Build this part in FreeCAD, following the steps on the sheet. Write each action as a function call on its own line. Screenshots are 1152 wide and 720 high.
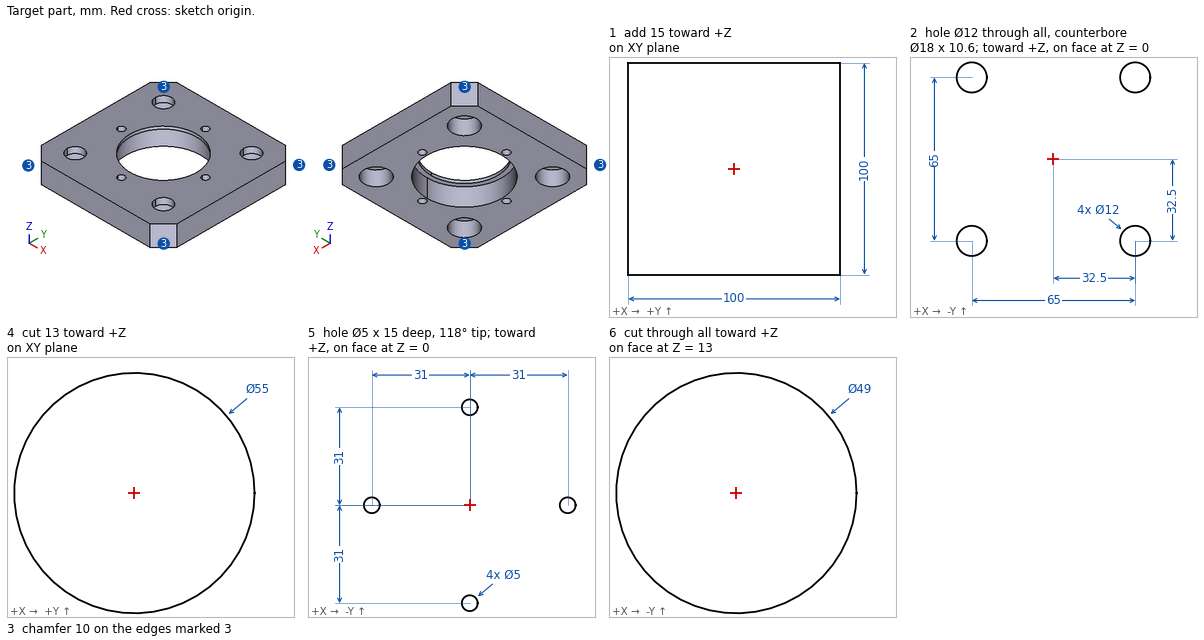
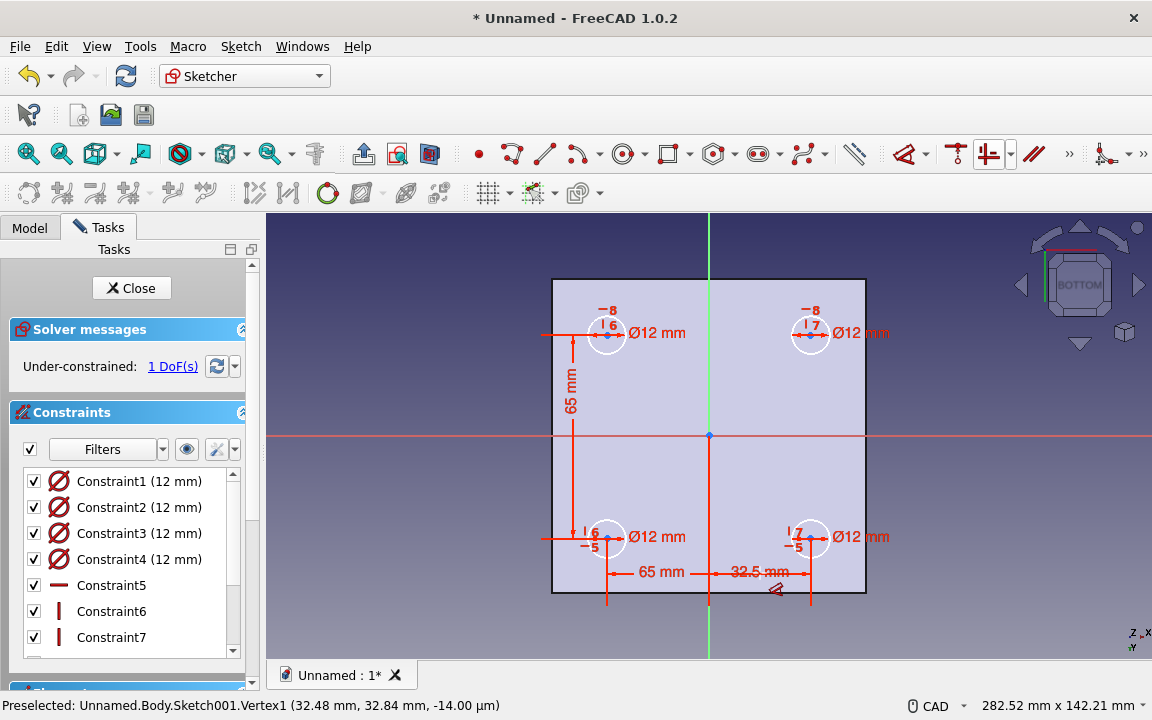
click(811, 539)
click(845, 487)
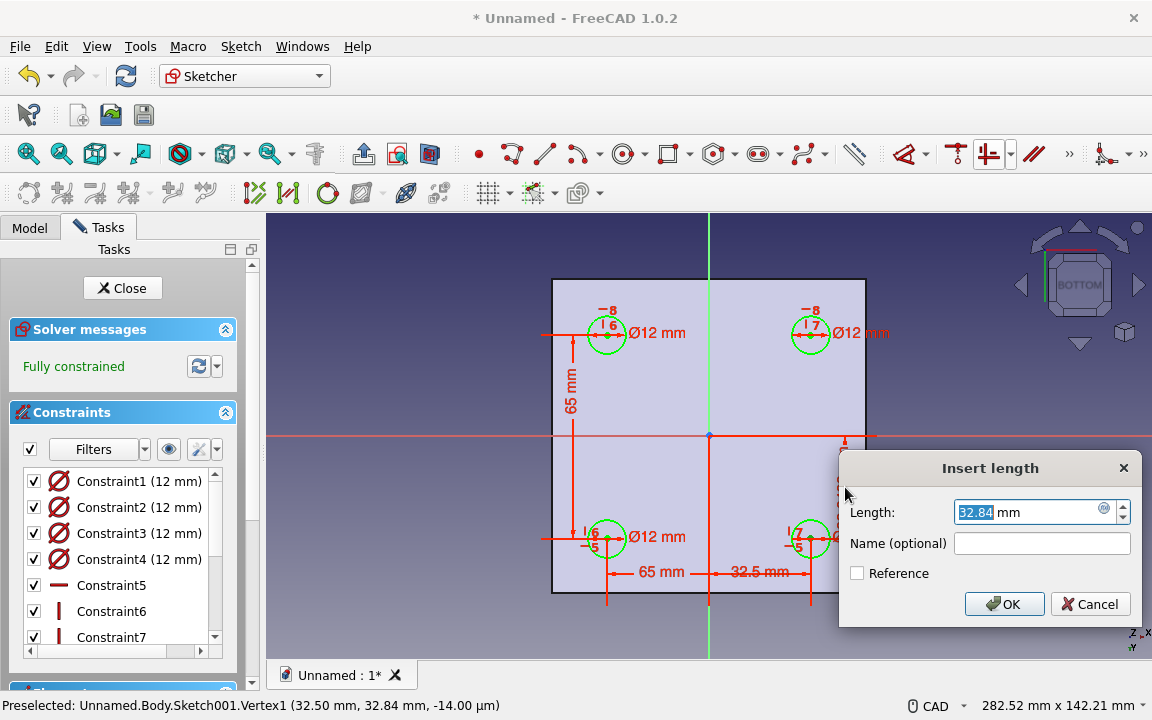
text(32.5)
key(Return)
key(Escape)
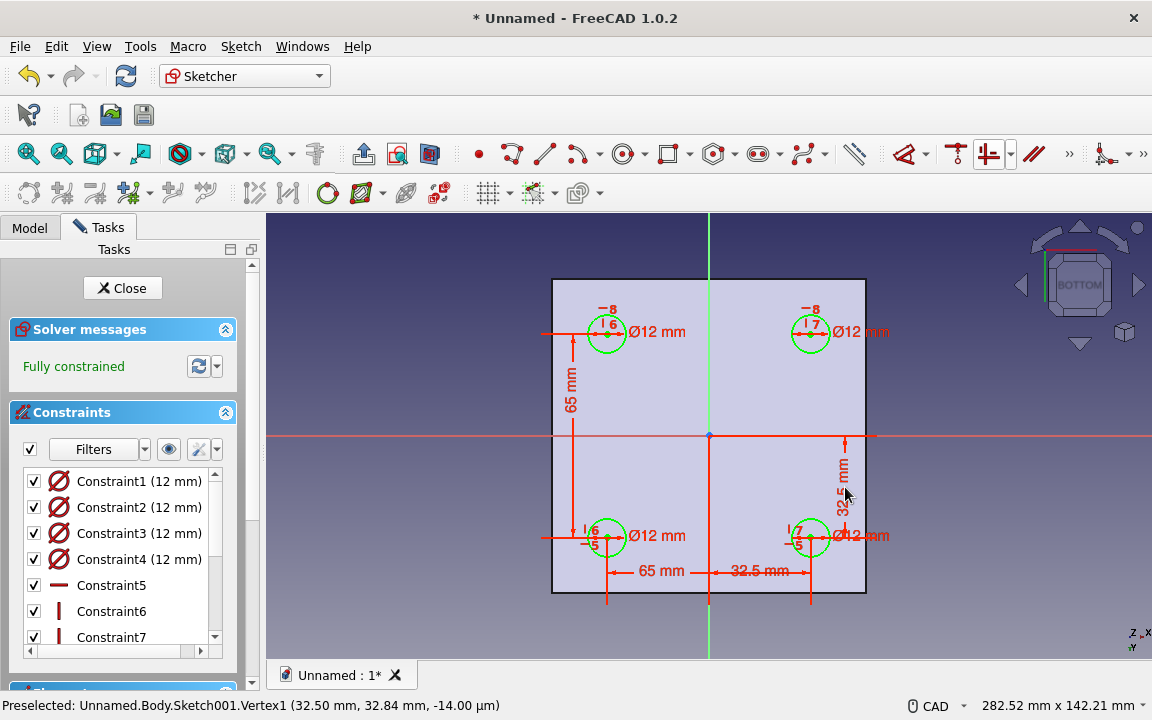
click(123, 288)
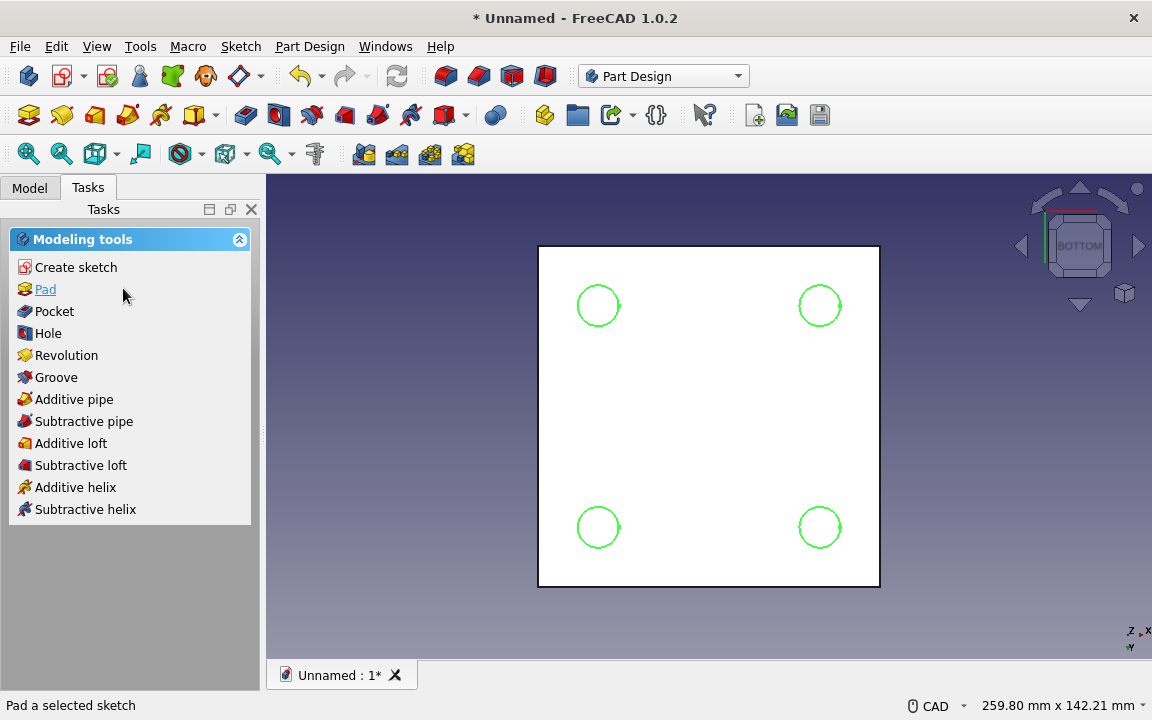
click(279, 116)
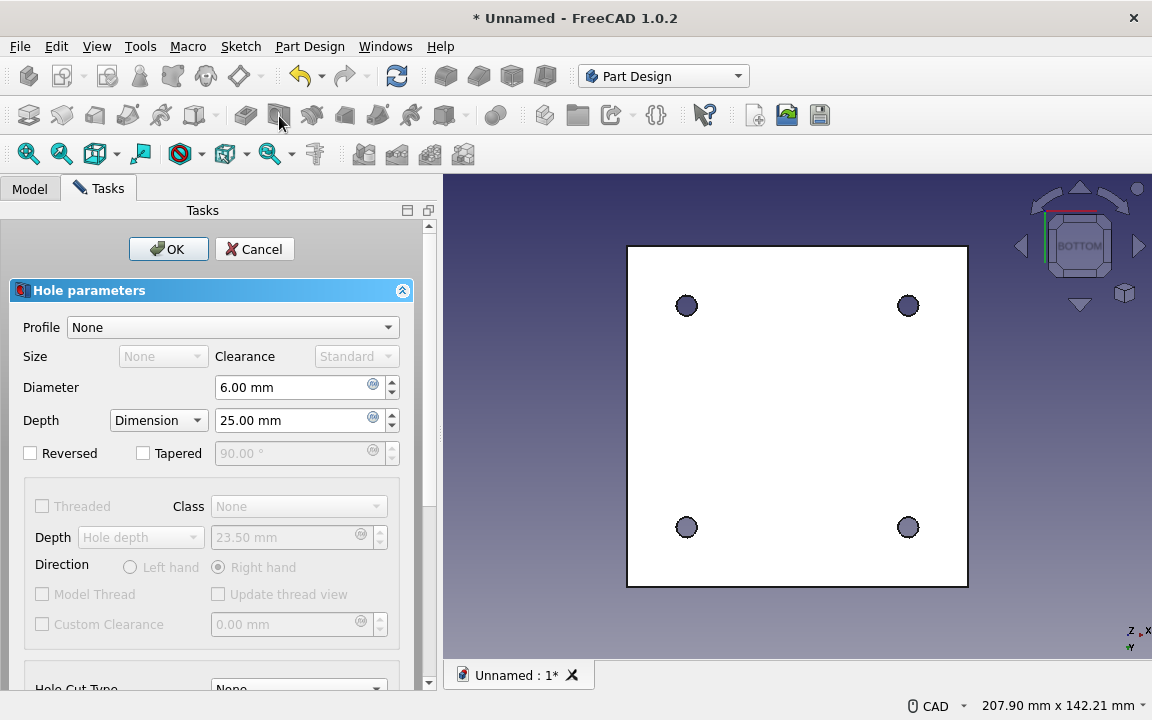
triple_click(300, 388)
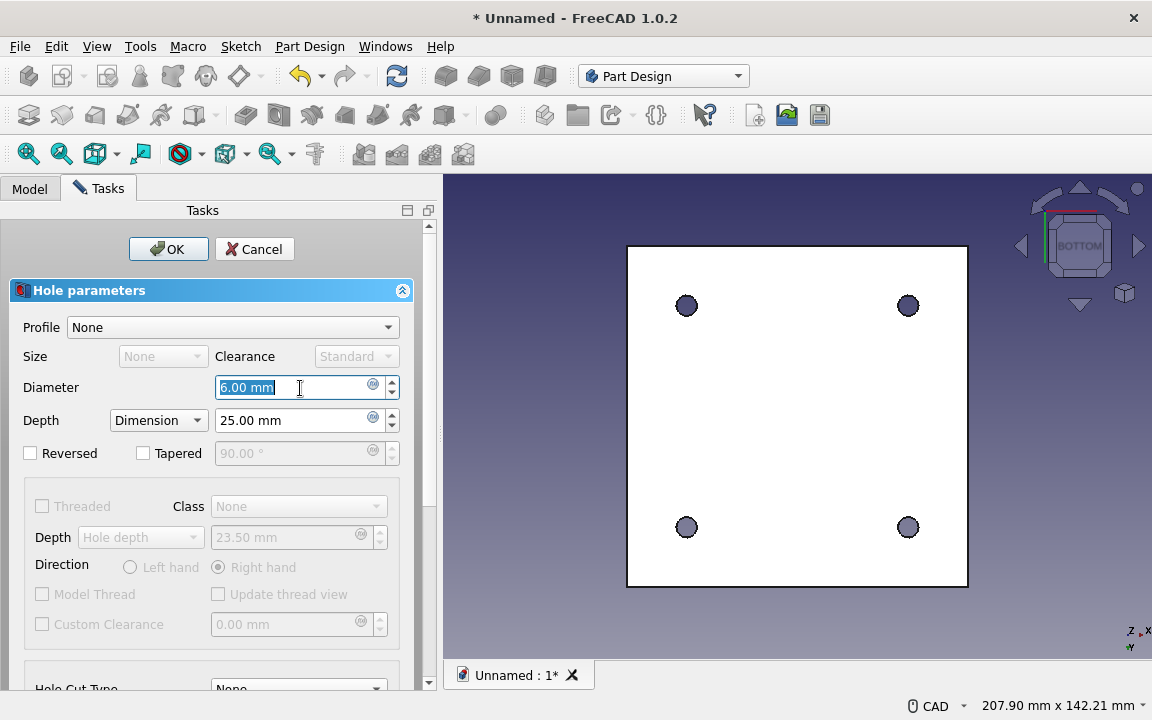
text(12)
key(Tab)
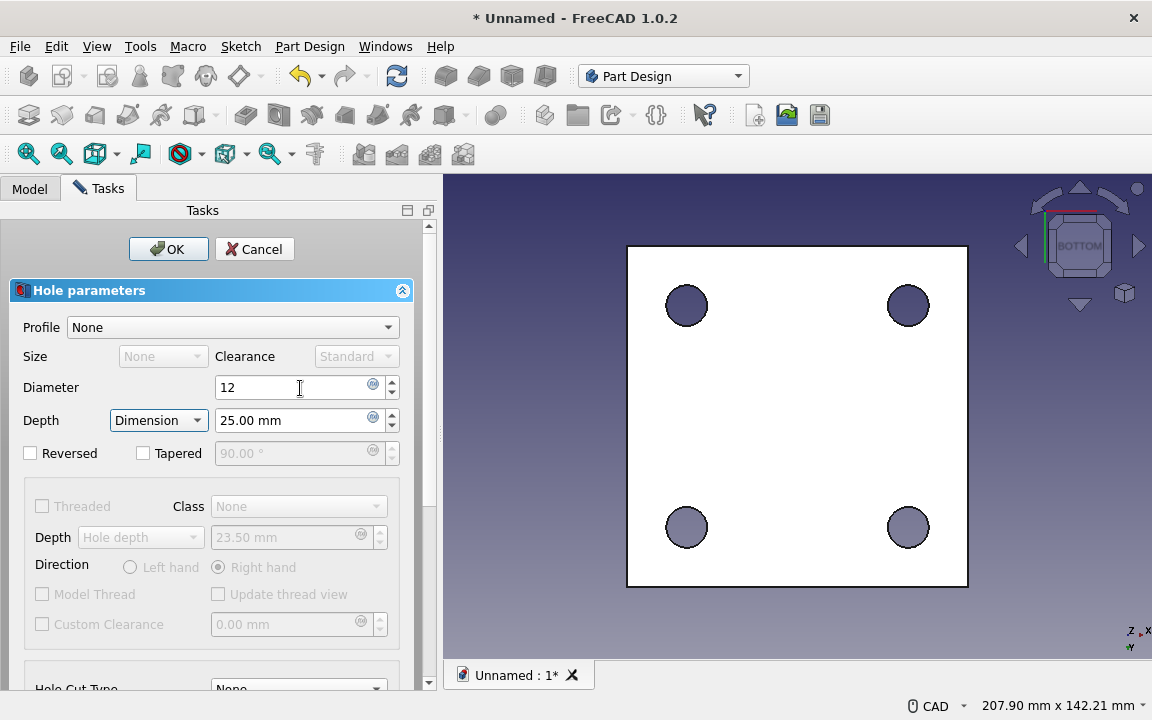
click(160, 420)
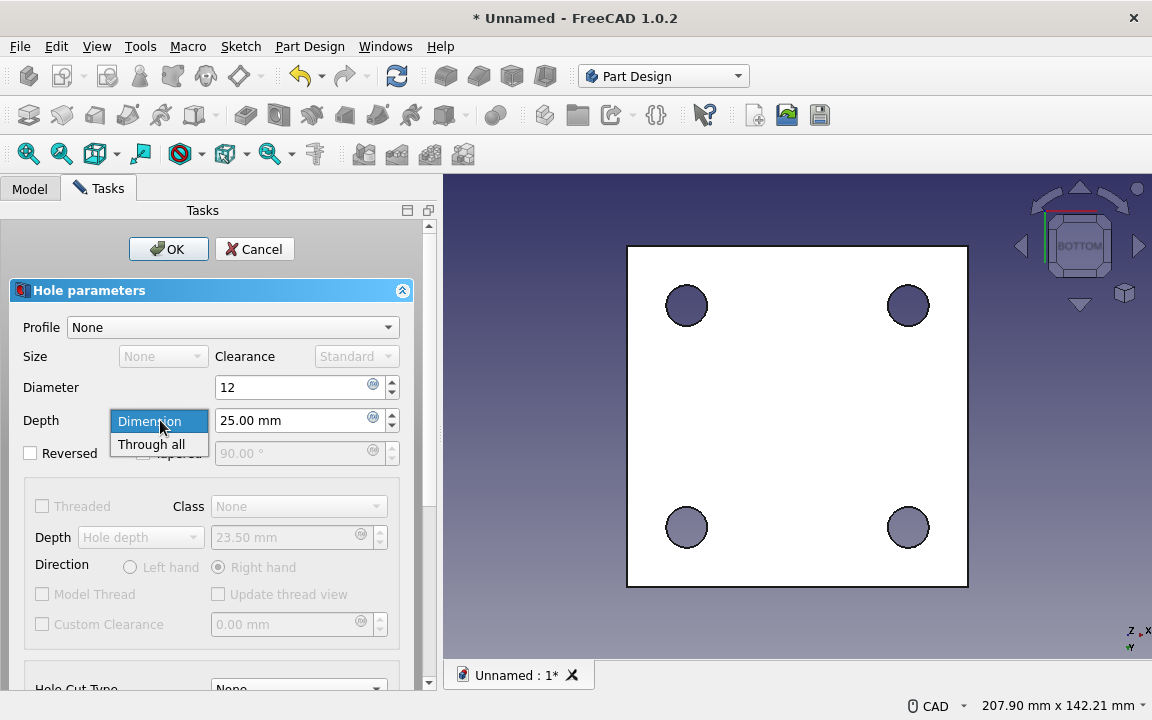
click(158, 444)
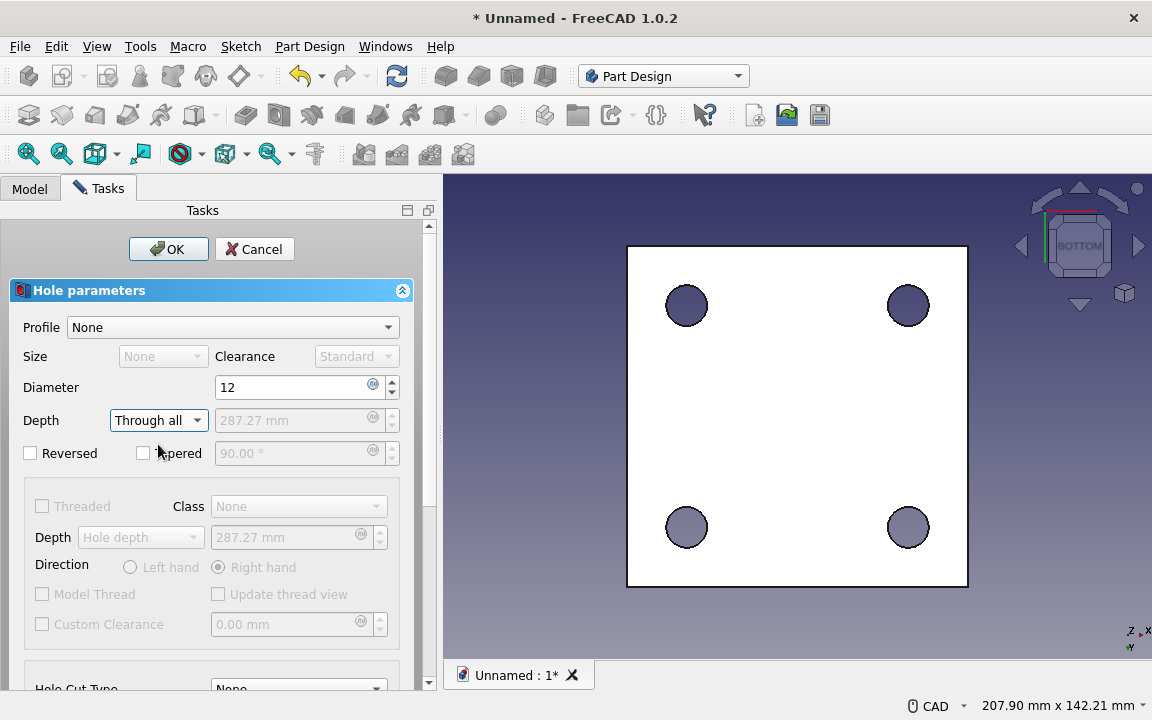
scroll(429, 455, down, 2)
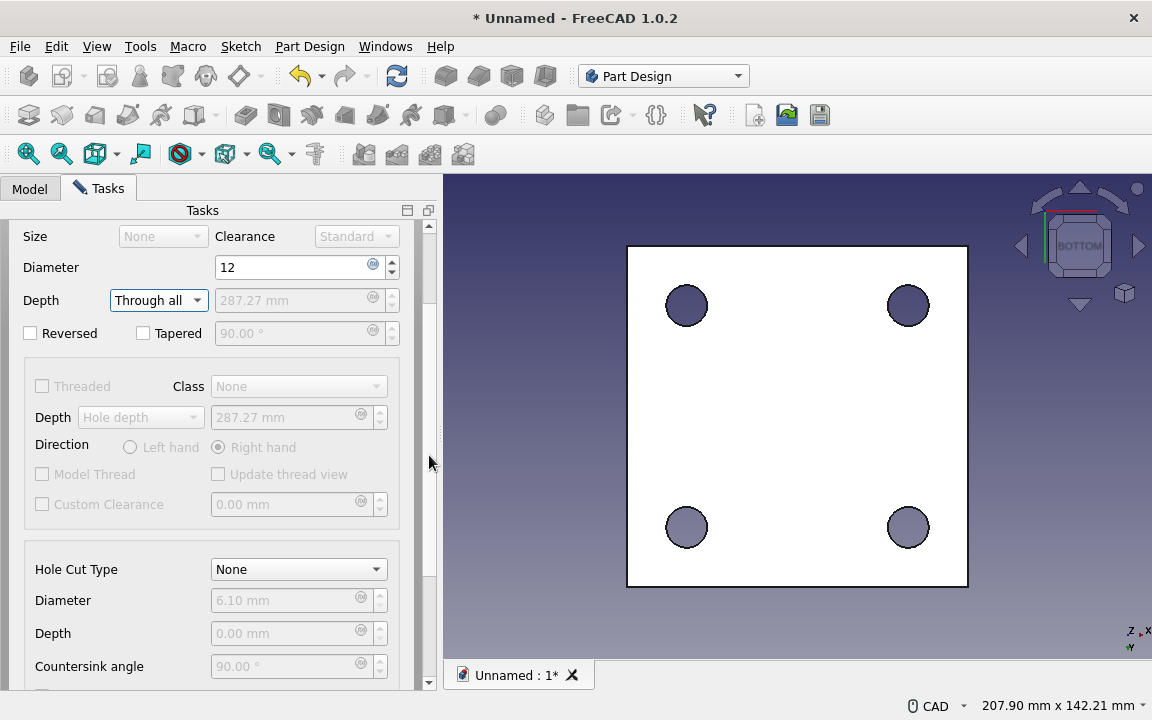
click(300, 570)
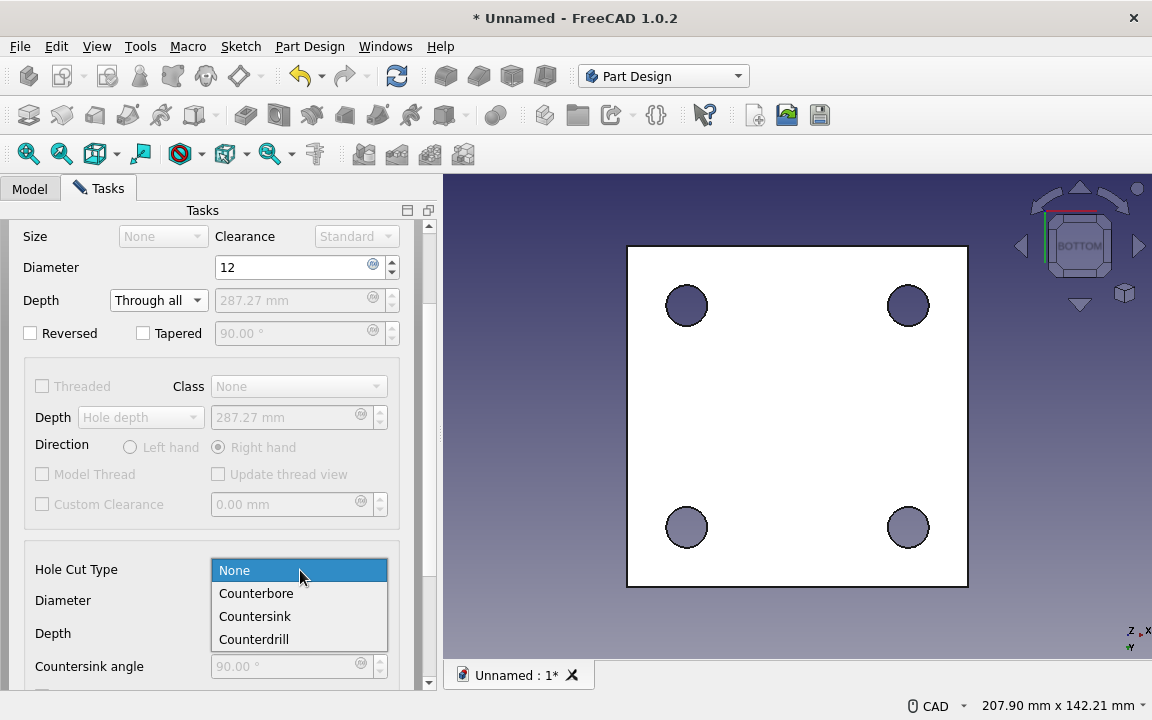
click(298, 594)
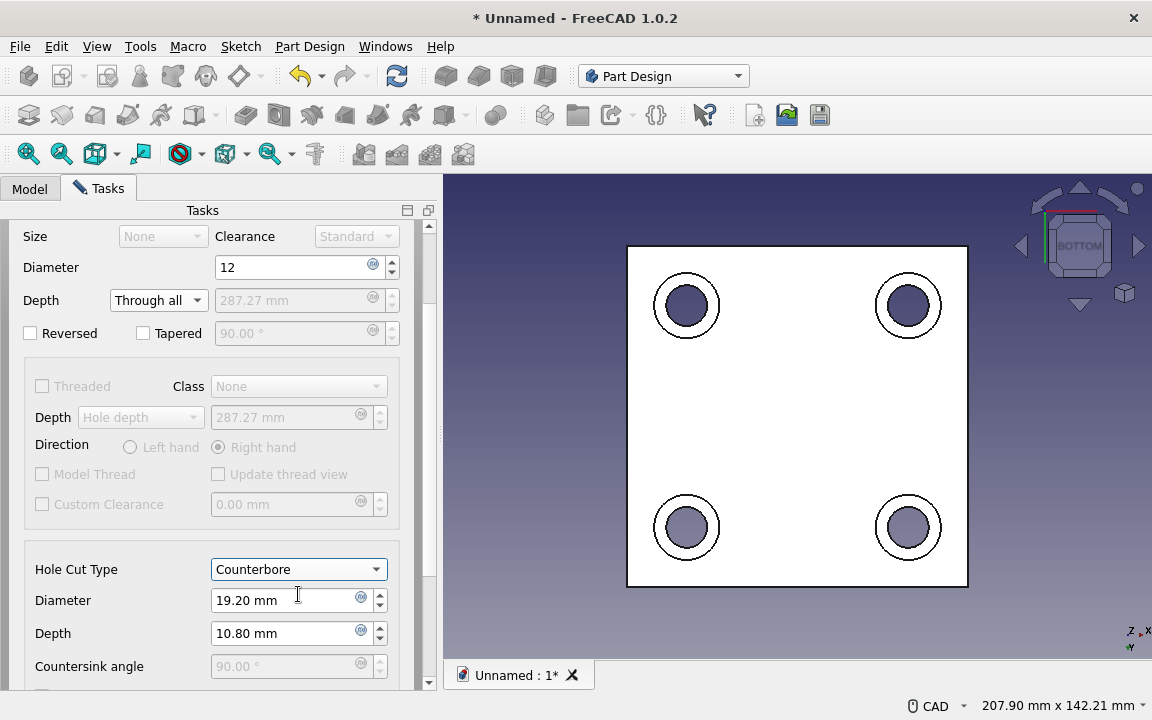
triple_click(292, 600)